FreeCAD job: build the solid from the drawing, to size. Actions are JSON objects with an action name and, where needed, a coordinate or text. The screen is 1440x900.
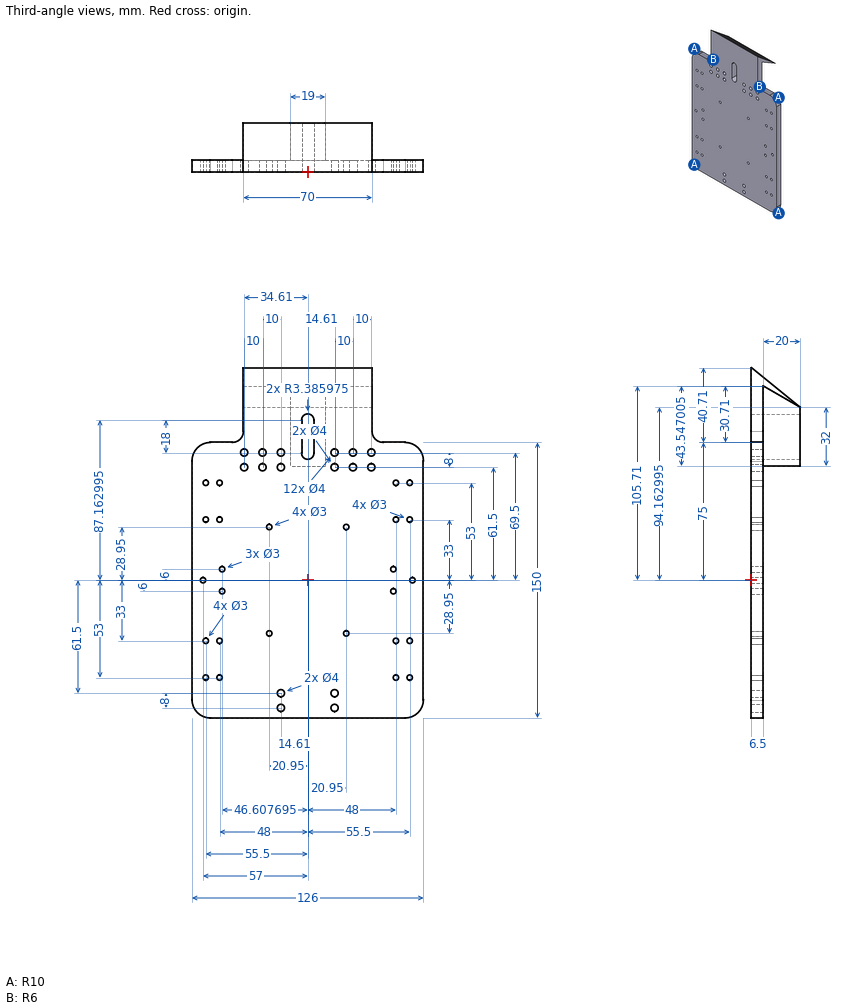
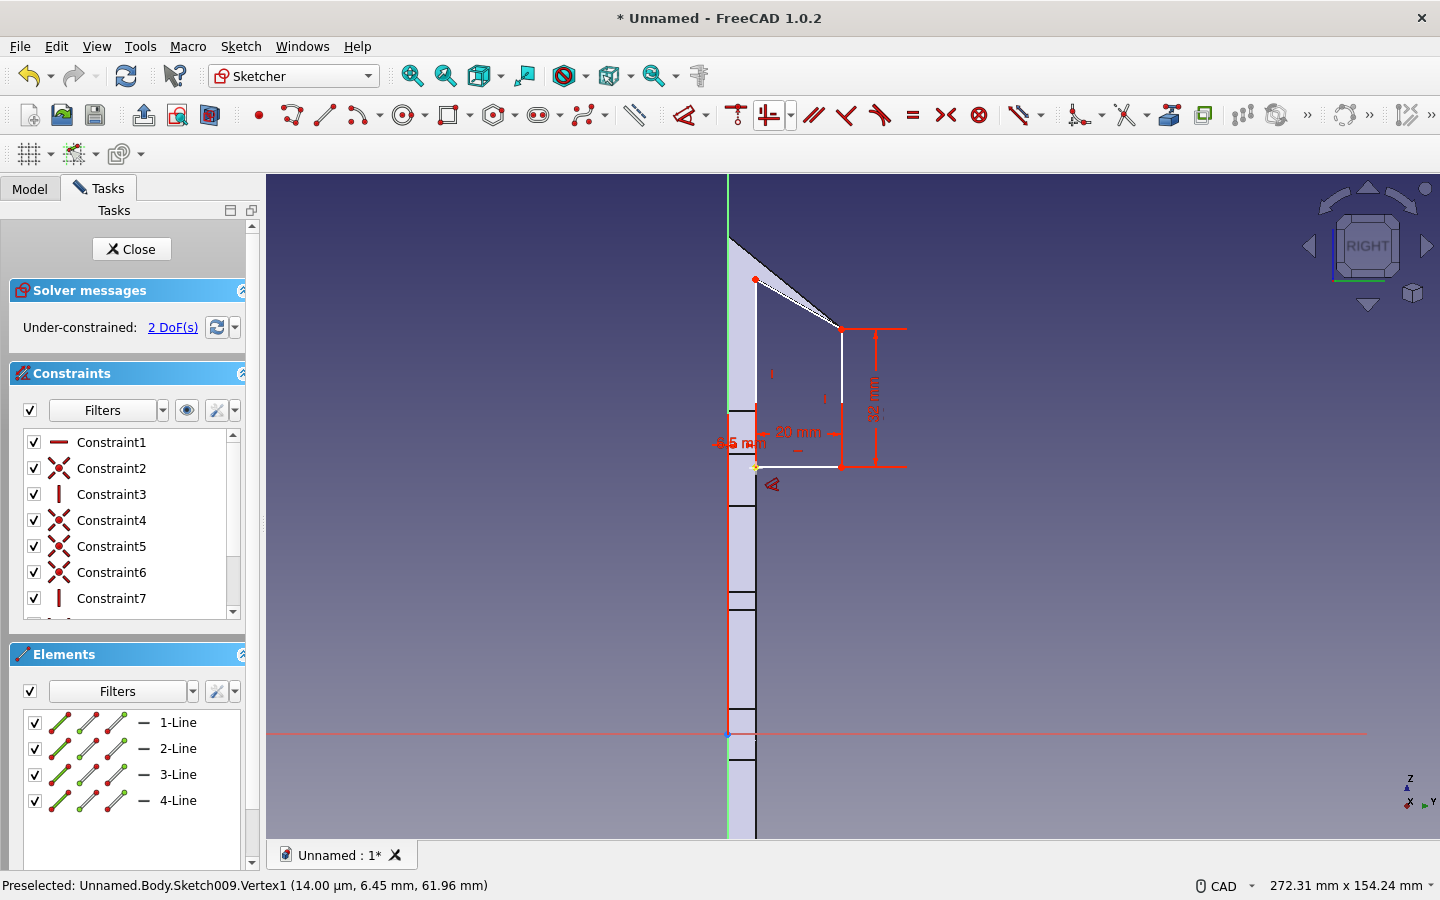
{"action": "left_click", "coordinate": [756, 279]}
{"action": "left_click", "coordinate": [694, 507]}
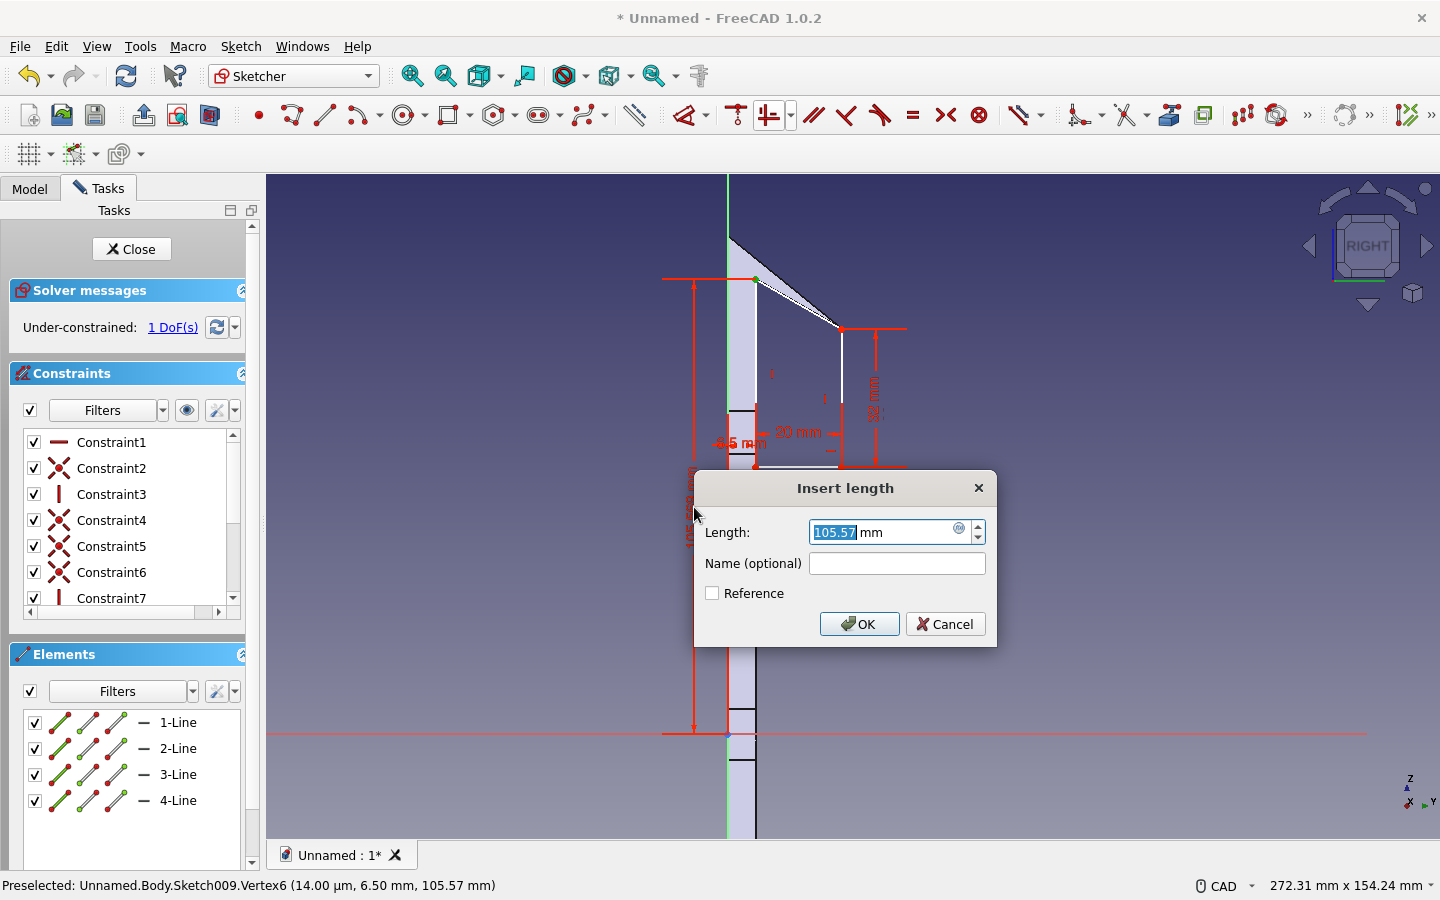
{"action": "type", "text": "105.71"}
{"action": "key", "text": "Return"}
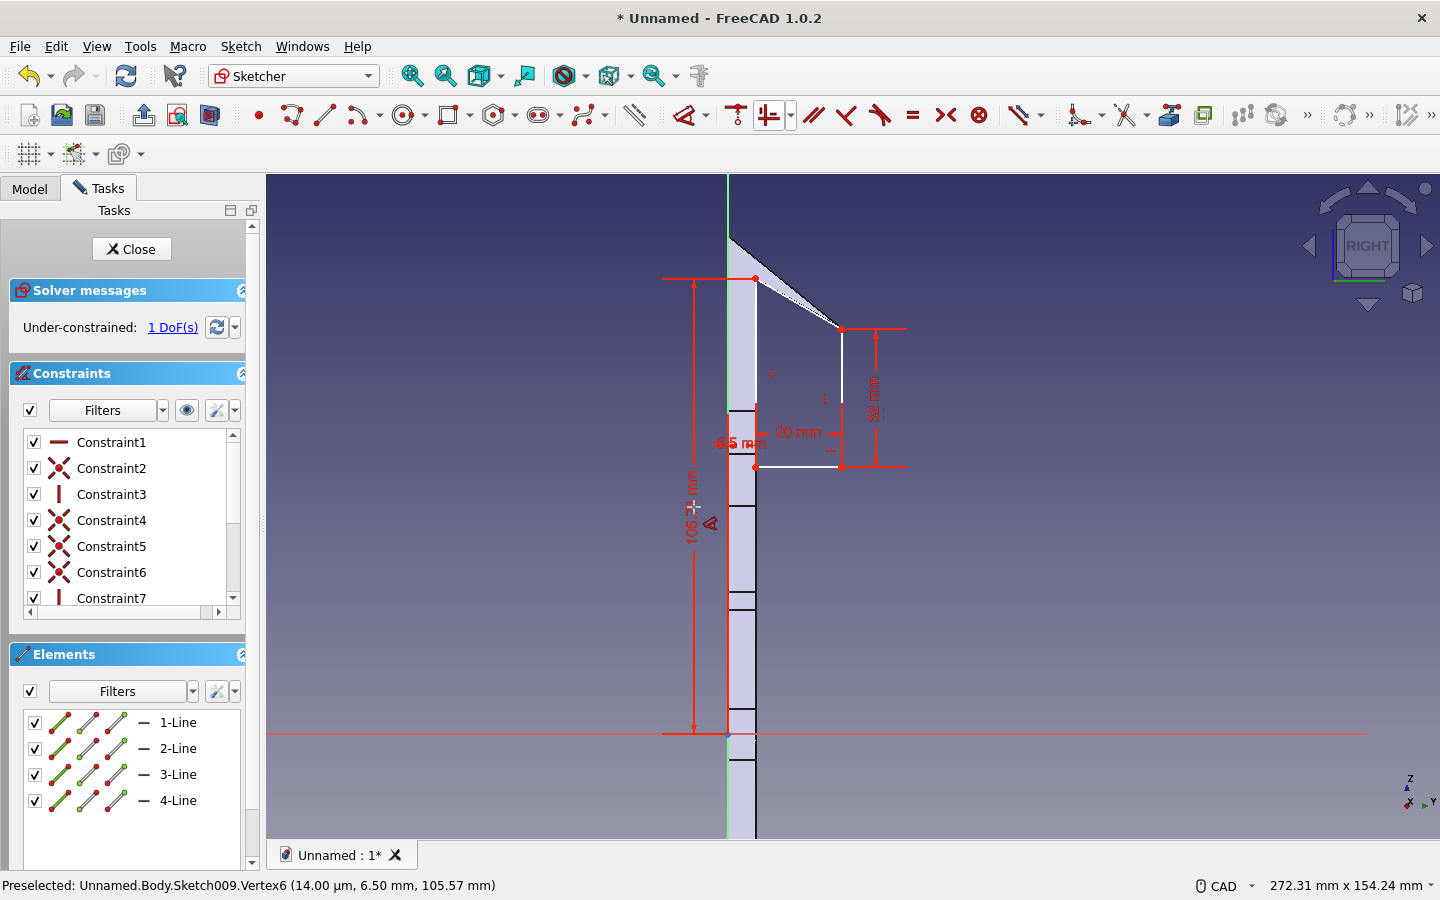
{"action": "left_click", "coordinate": [756, 335]}
{"action": "left_click", "coordinate": [790, 373]}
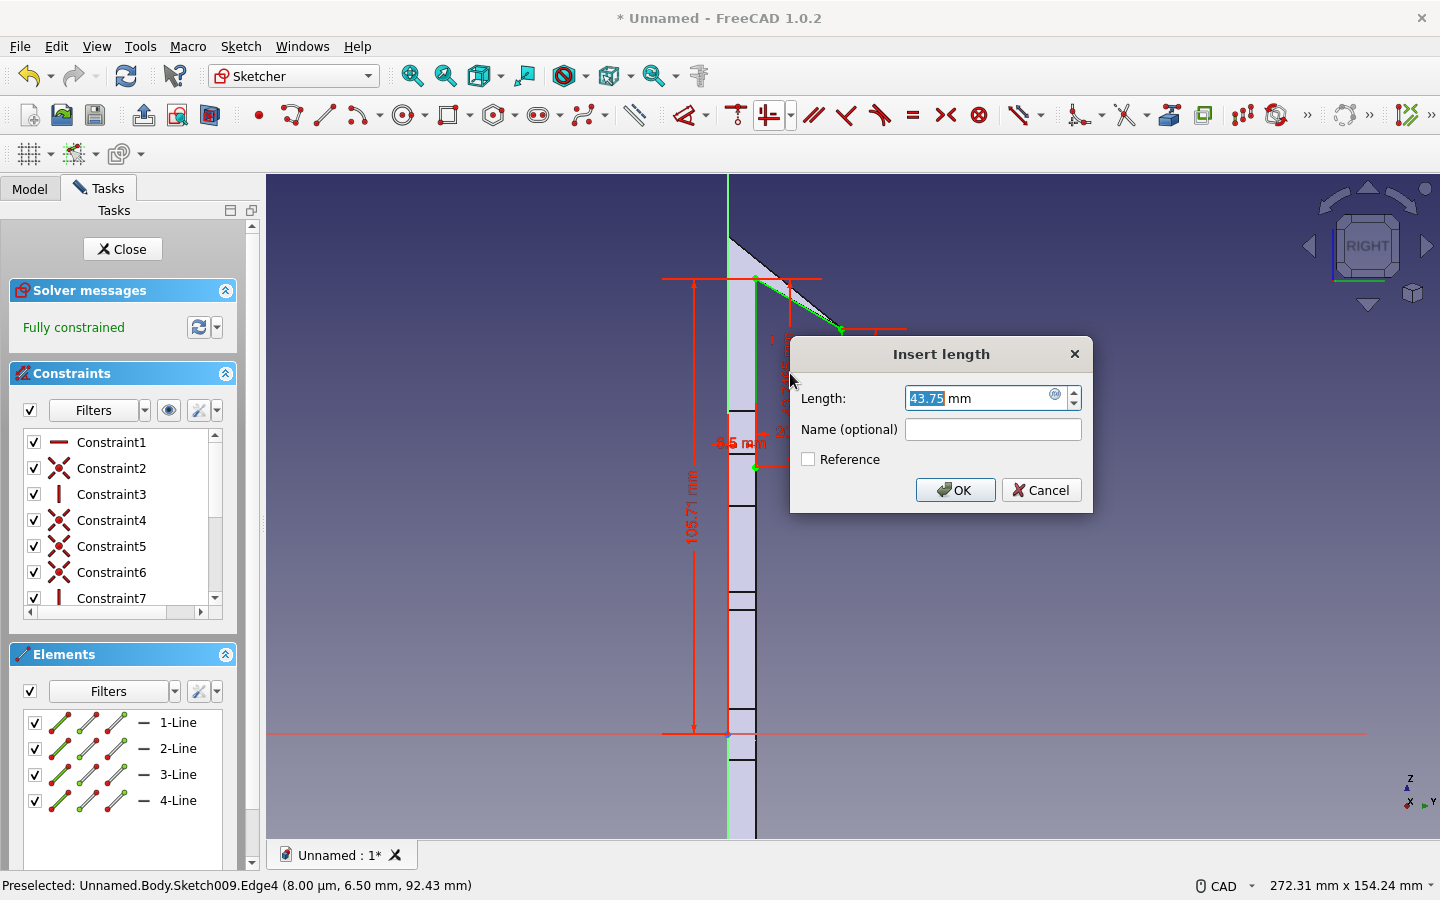
{"action": "type", "text": "43.547005"}
{"action": "key", "text": "Return"}
{"action": "key", "text": "Escape"}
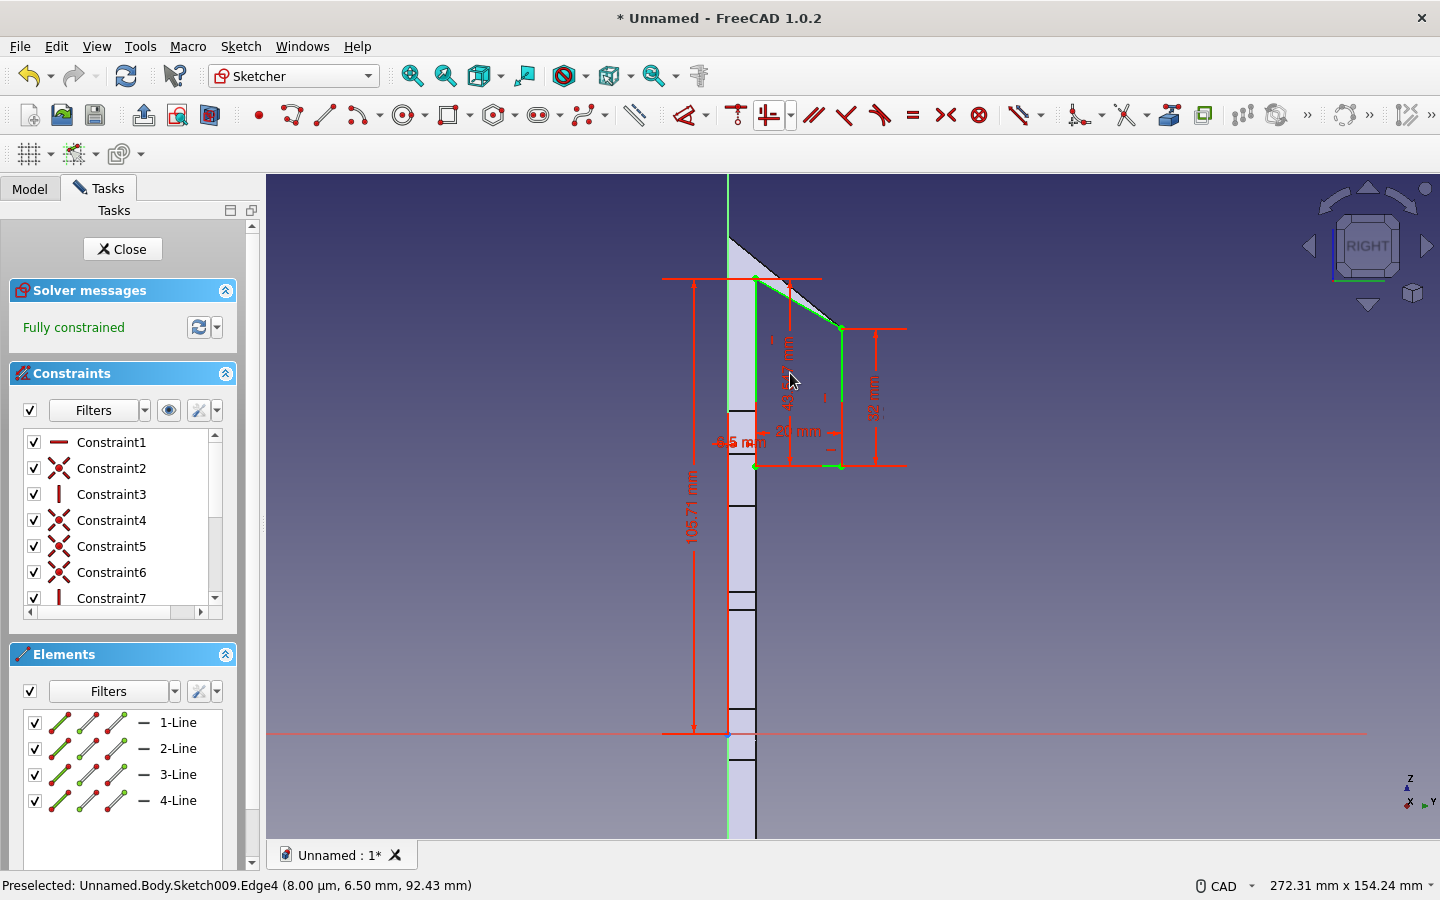
{"action": "left_click", "coordinate": [123, 249]}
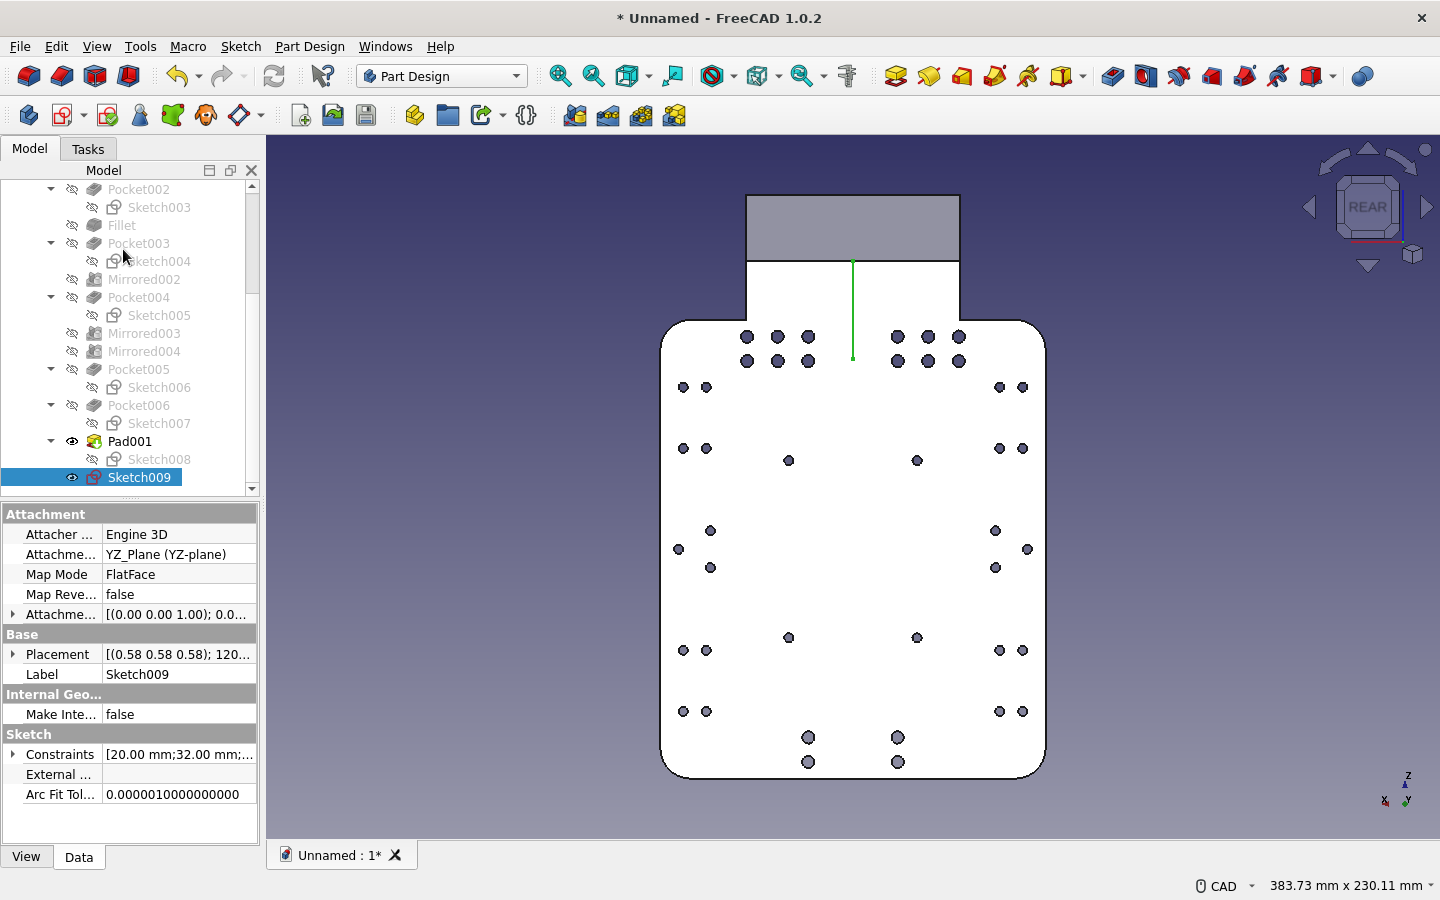
{"action": "left_click", "coordinate": [896, 76]}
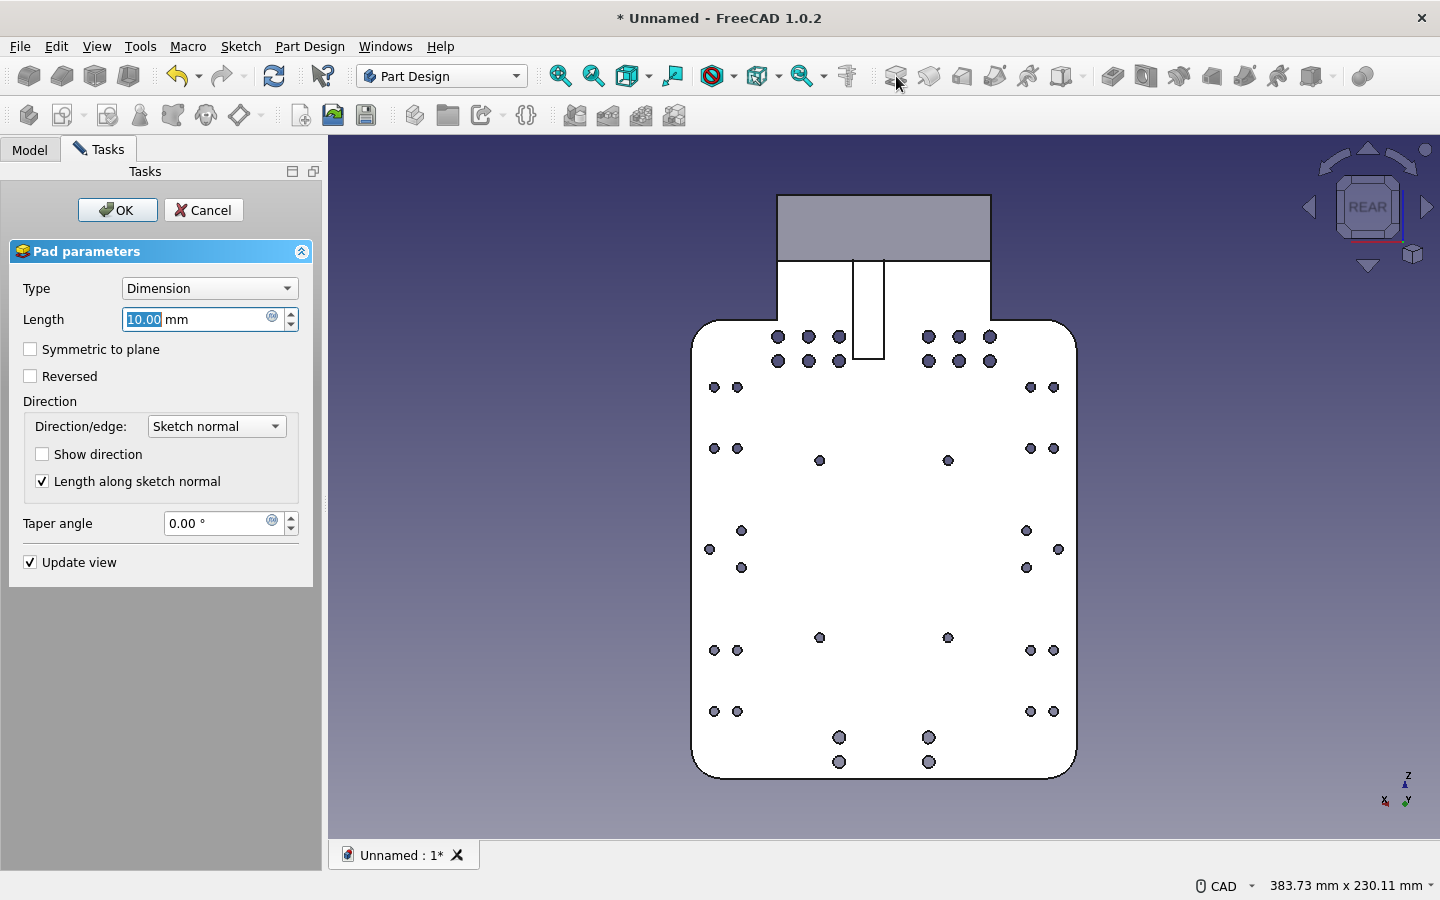
{"action": "type", "text": "19"}
{"action": "key", "text": "Tab"}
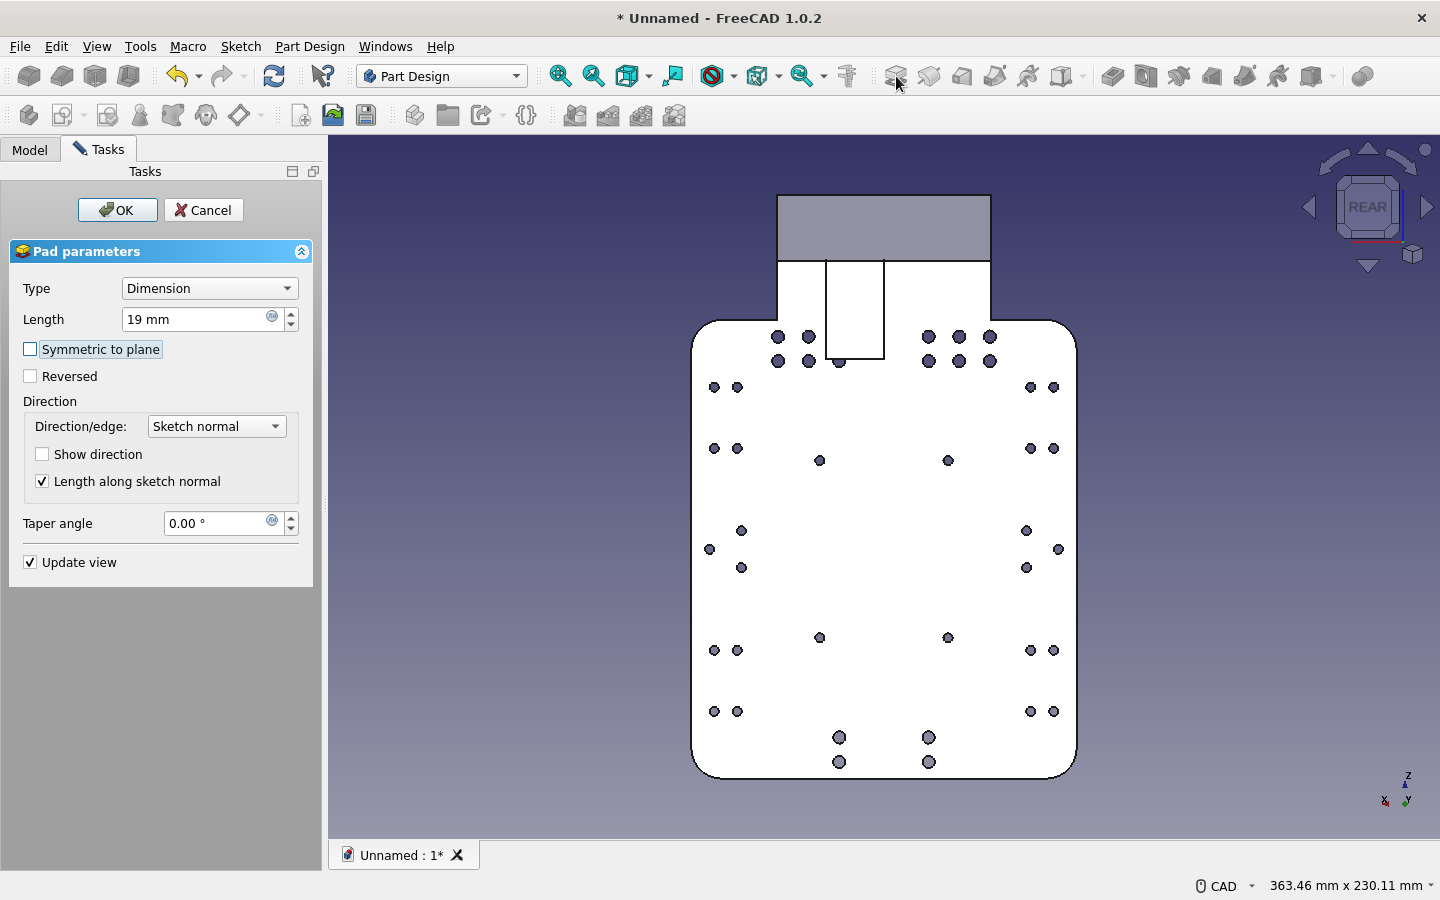
{"action": "left_click", "coordinate": [31, 349]}